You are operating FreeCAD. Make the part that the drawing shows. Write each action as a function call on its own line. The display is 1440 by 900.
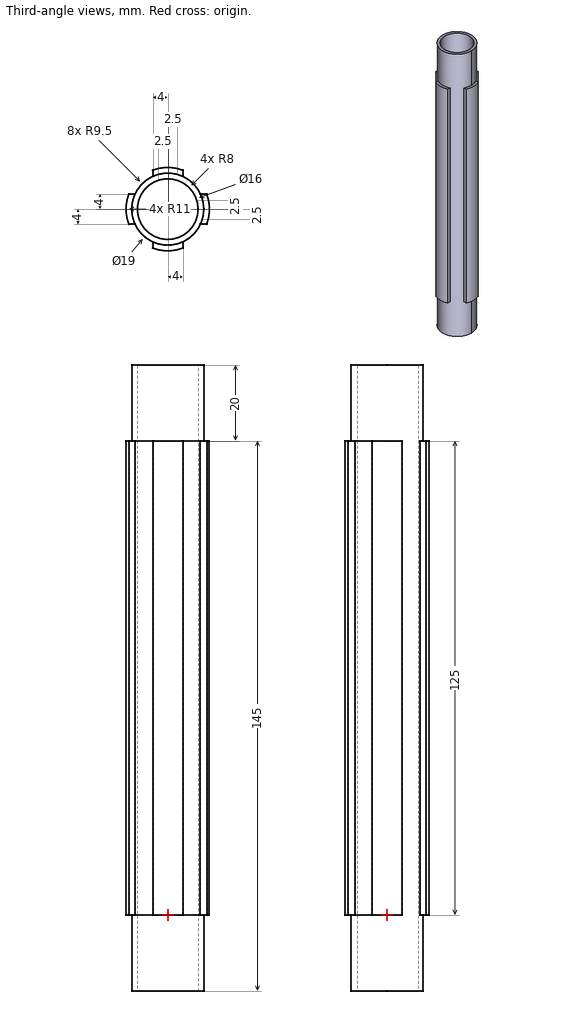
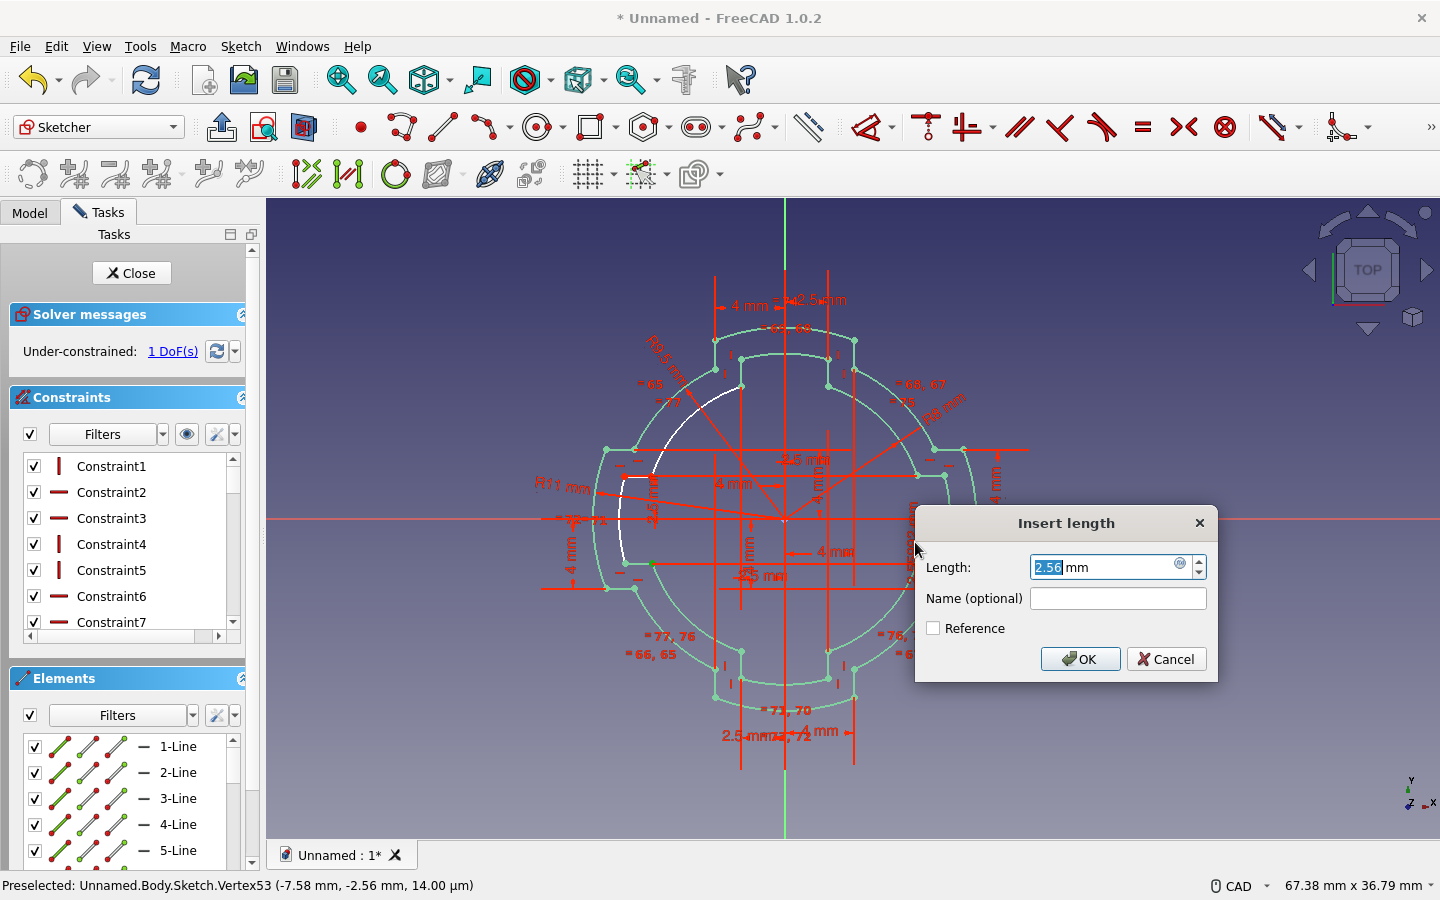
text(2.5)
key(Return)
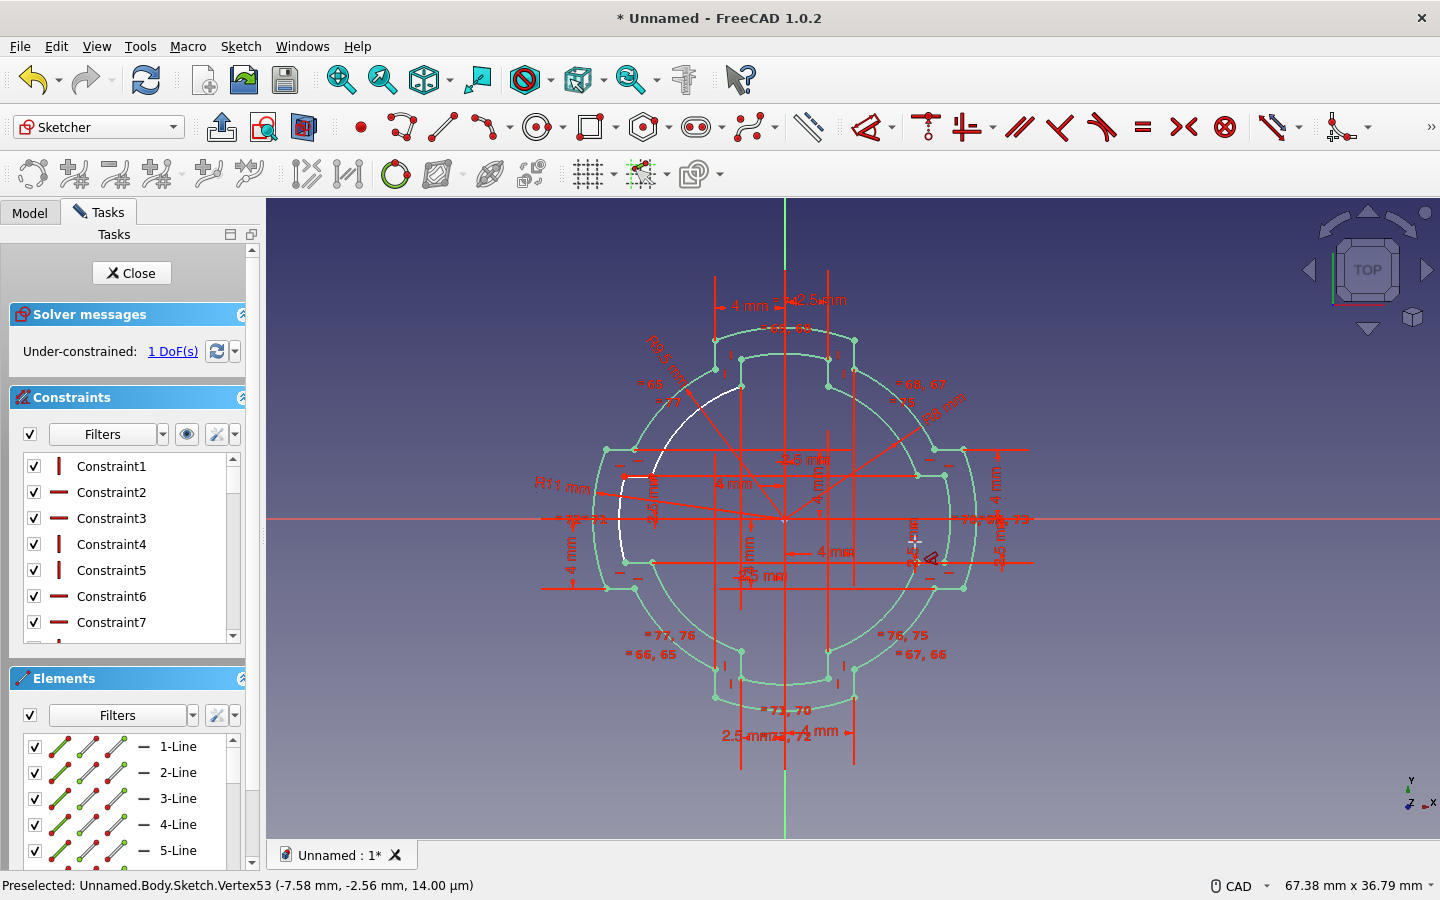
click(625, 477)
click(891, 498)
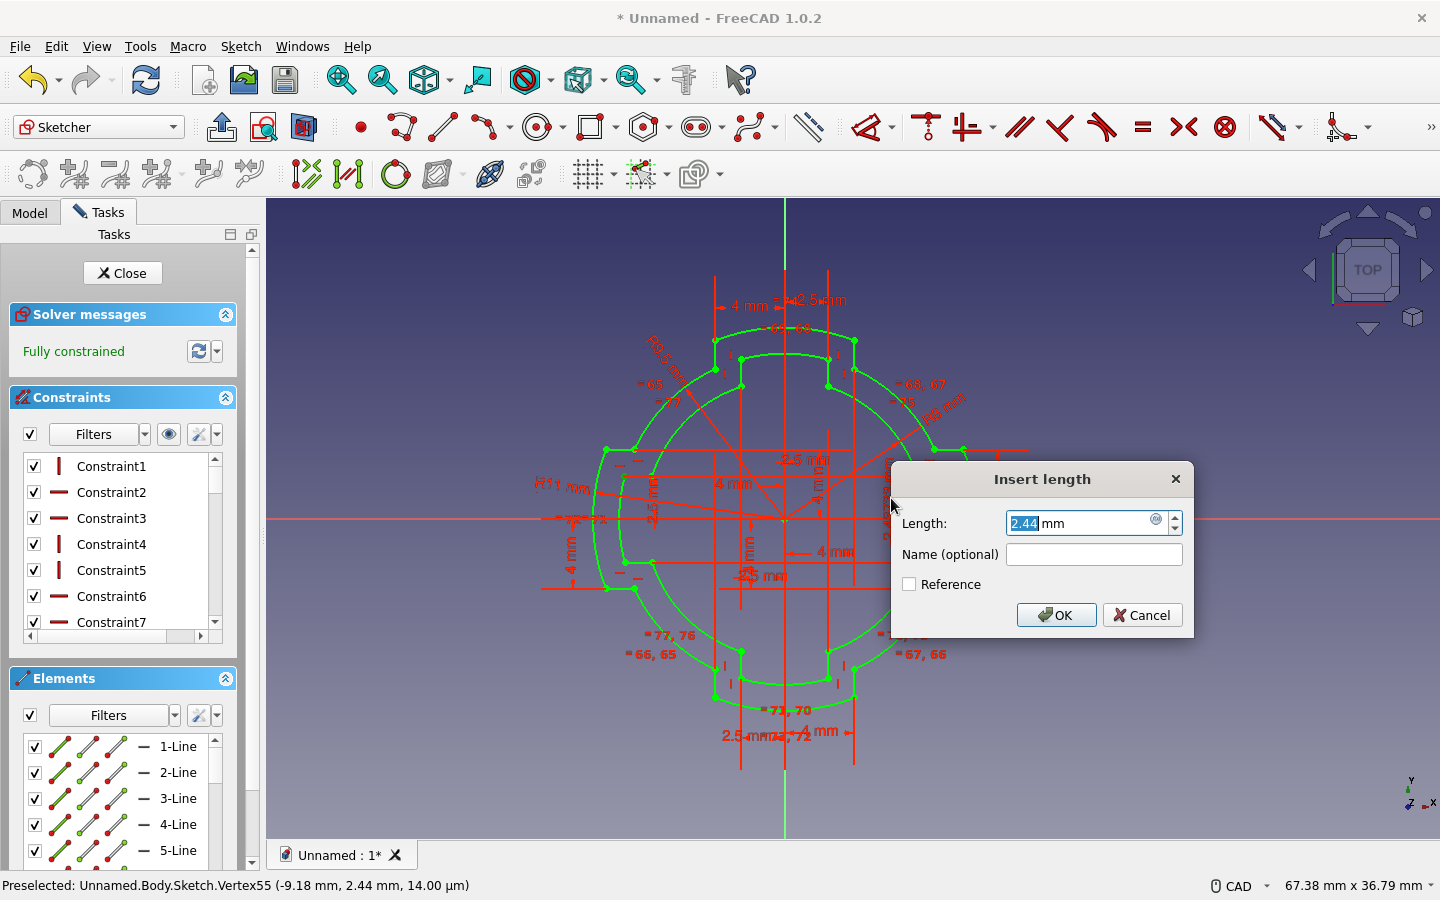
text(2.5)
key(Return)
key(Escape)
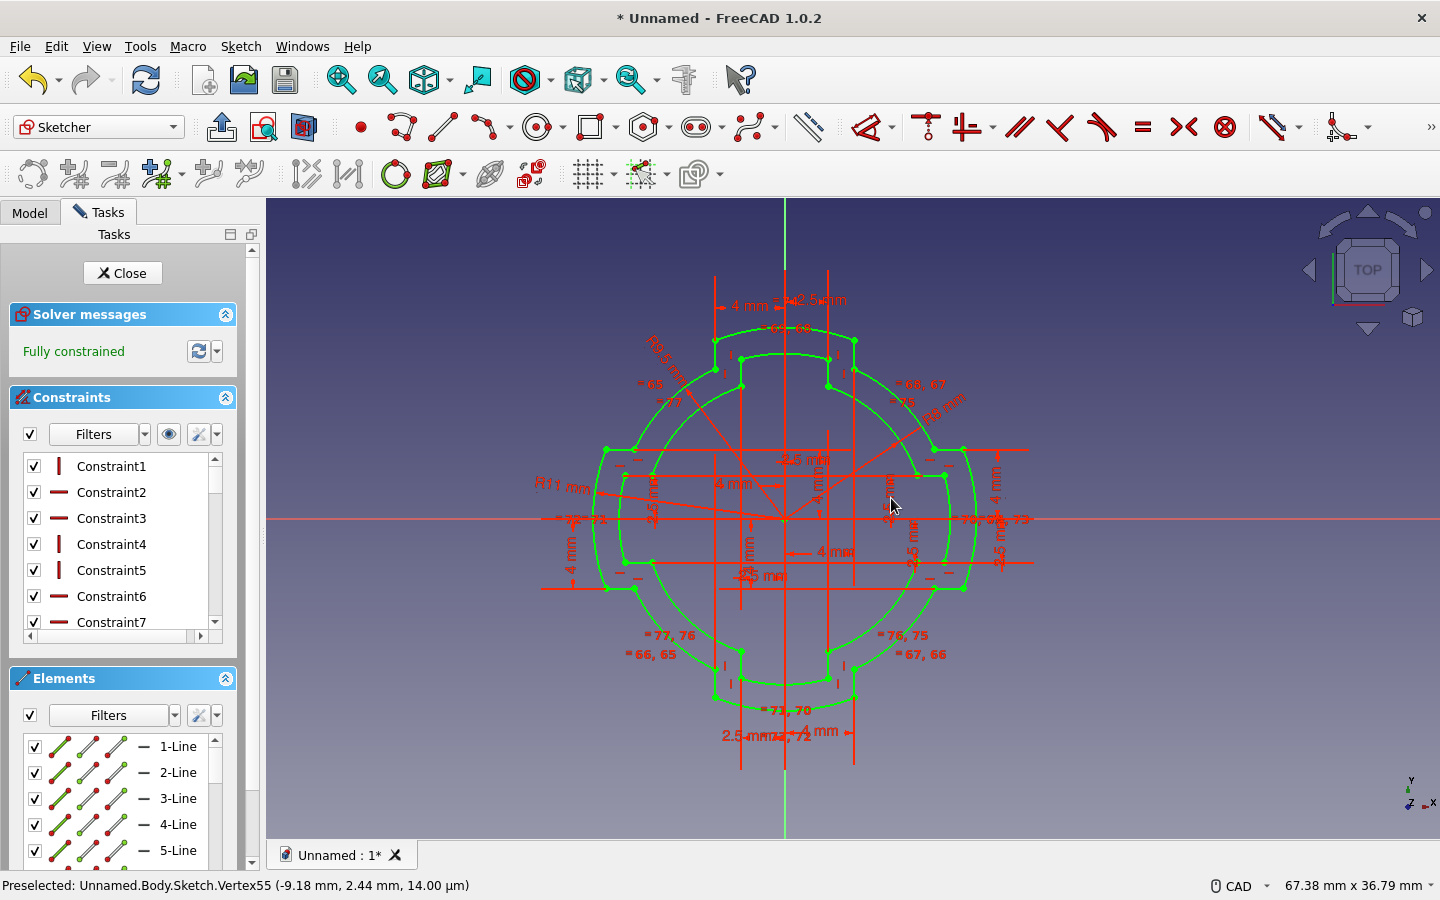
click(123, 273)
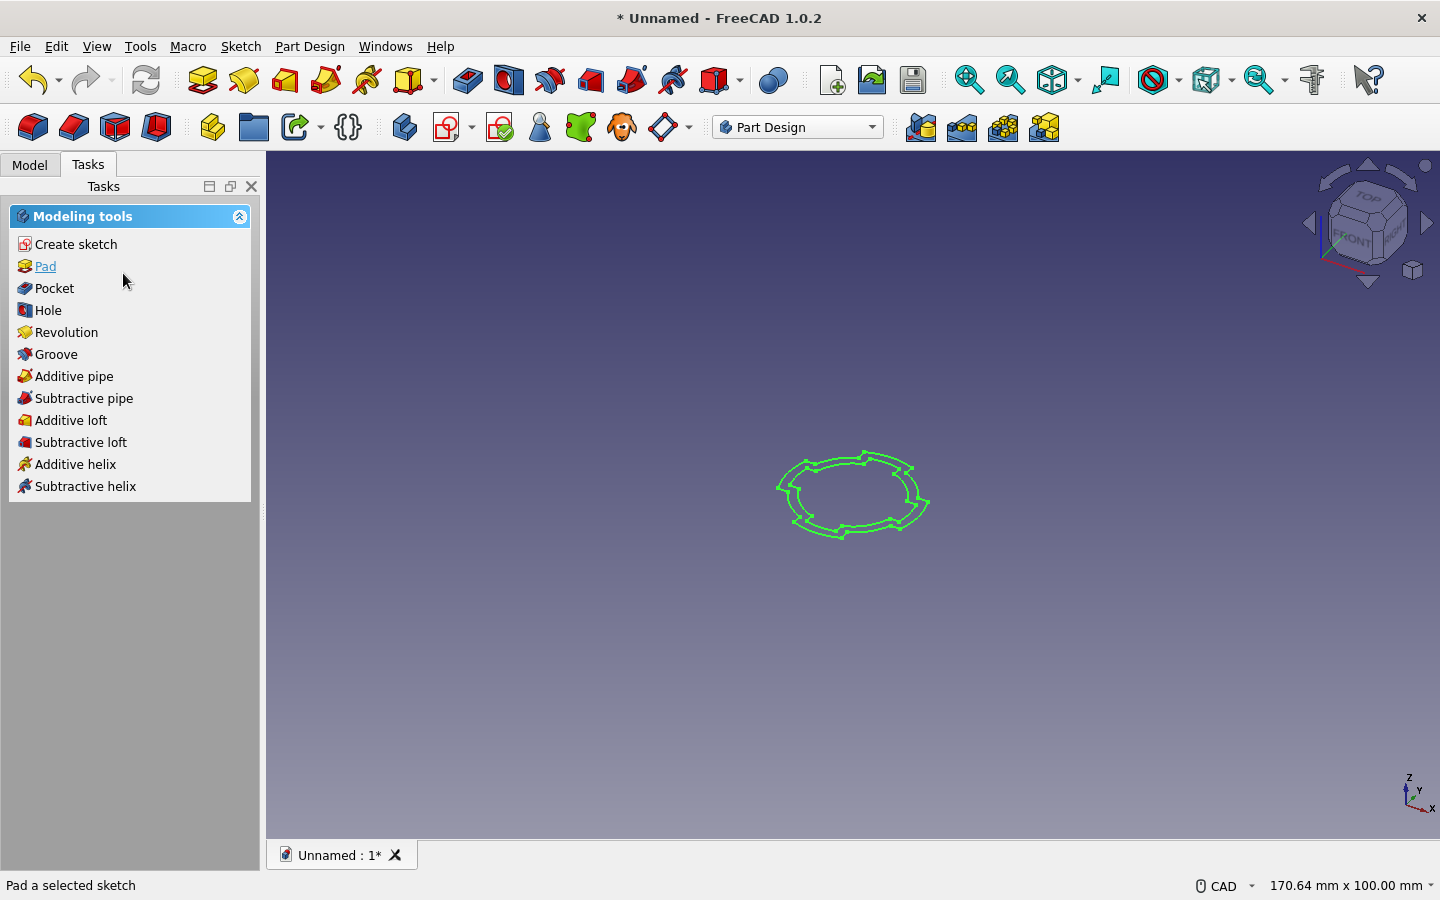
click(203, 80)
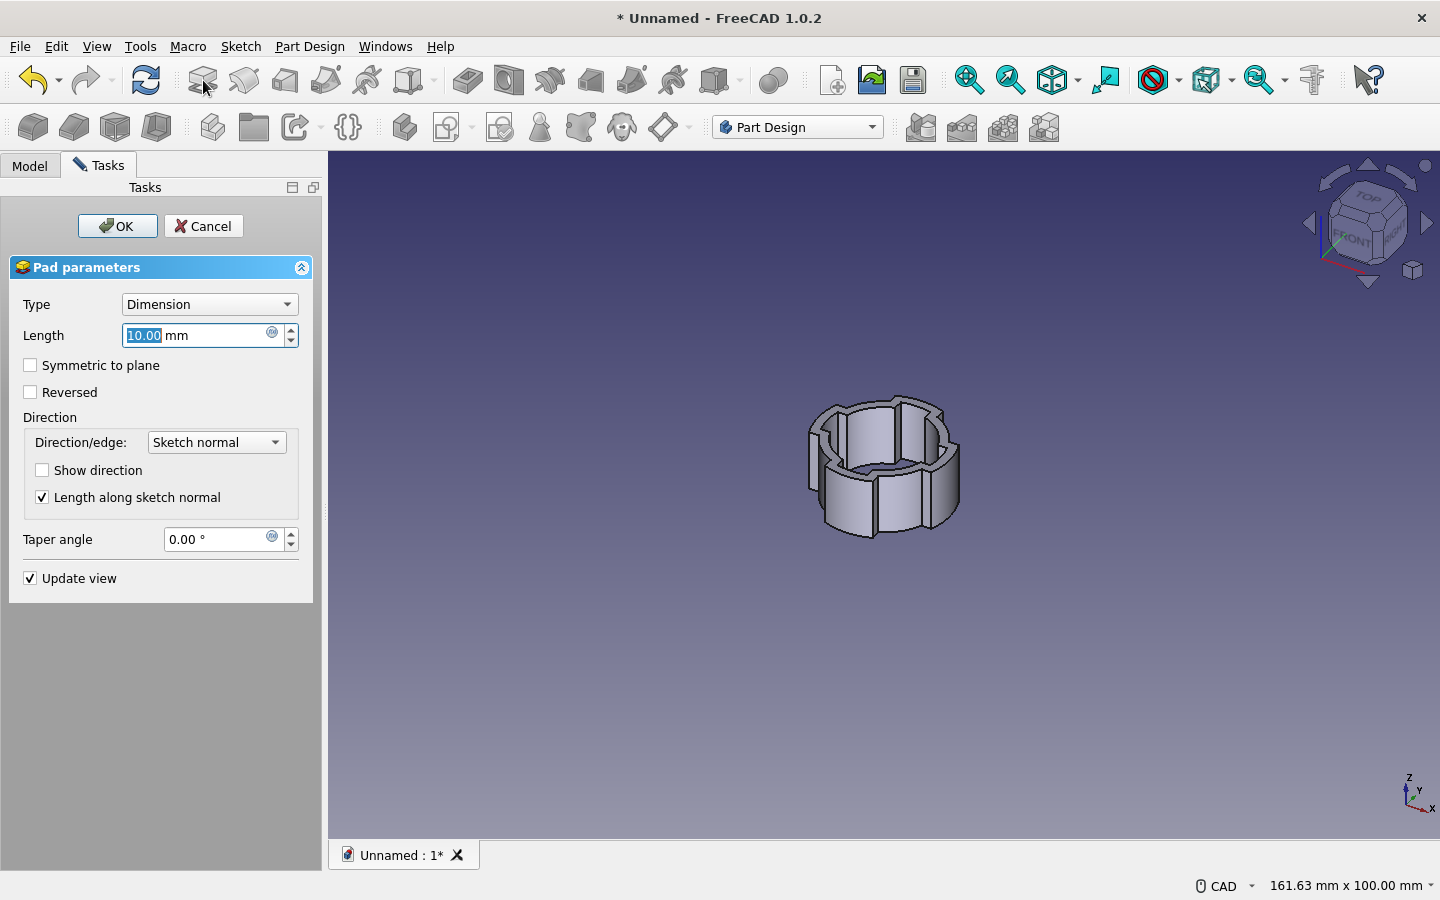
text(125)
key(Tab)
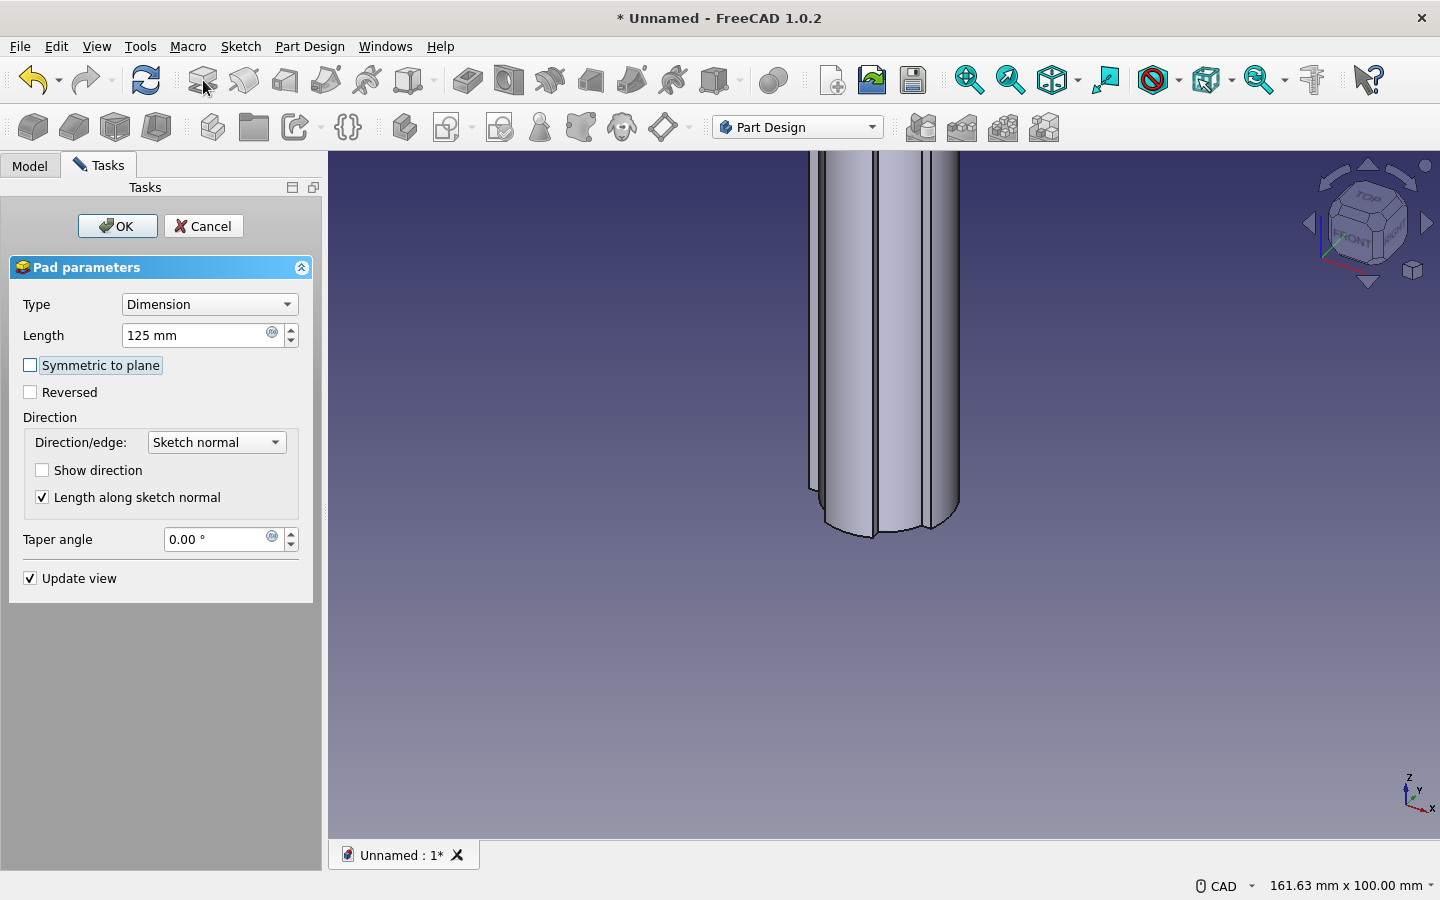
click(118, 226)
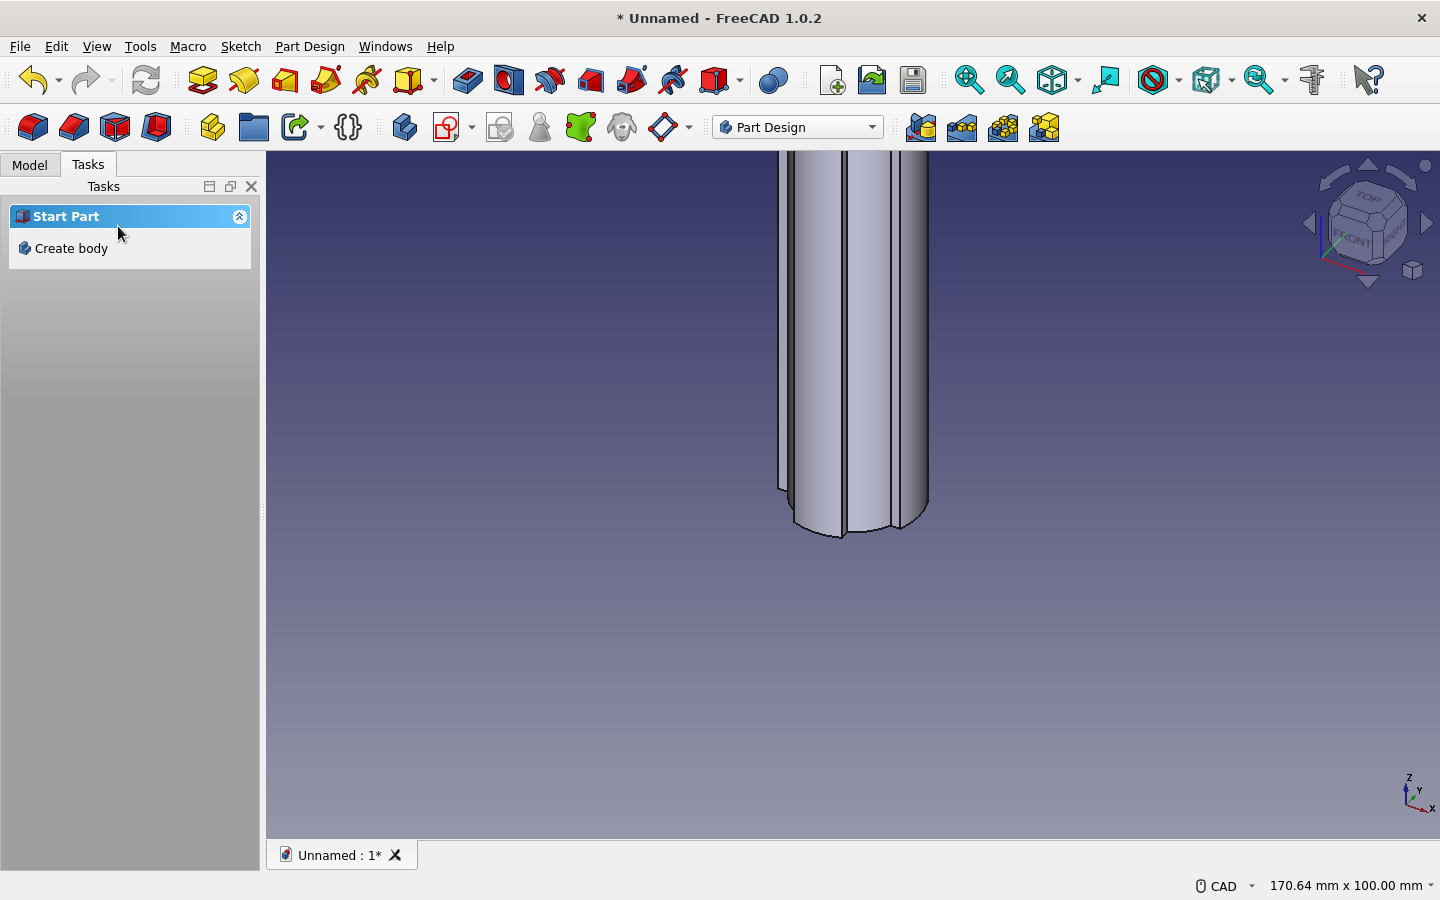
click(970, 80)